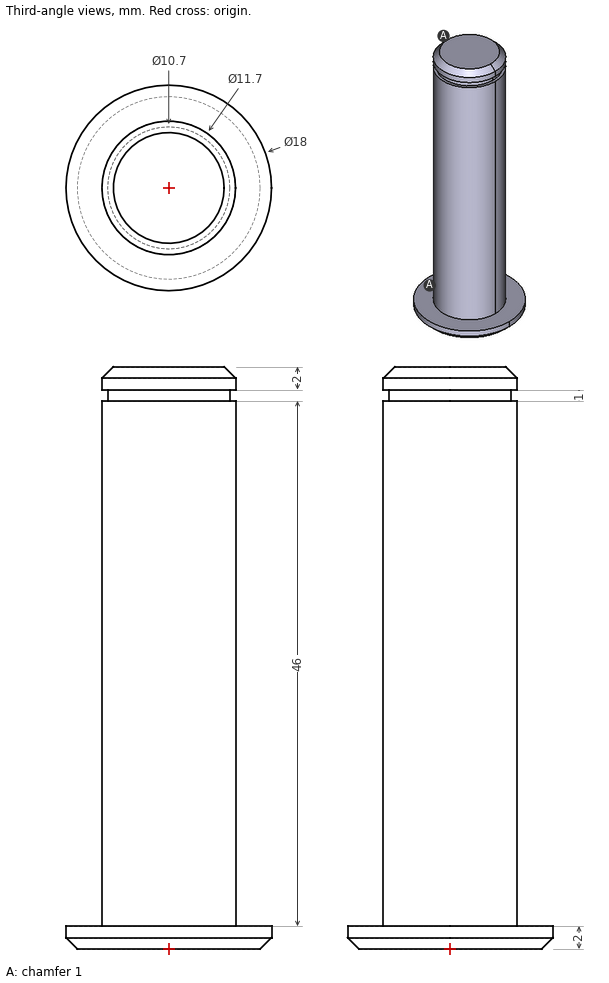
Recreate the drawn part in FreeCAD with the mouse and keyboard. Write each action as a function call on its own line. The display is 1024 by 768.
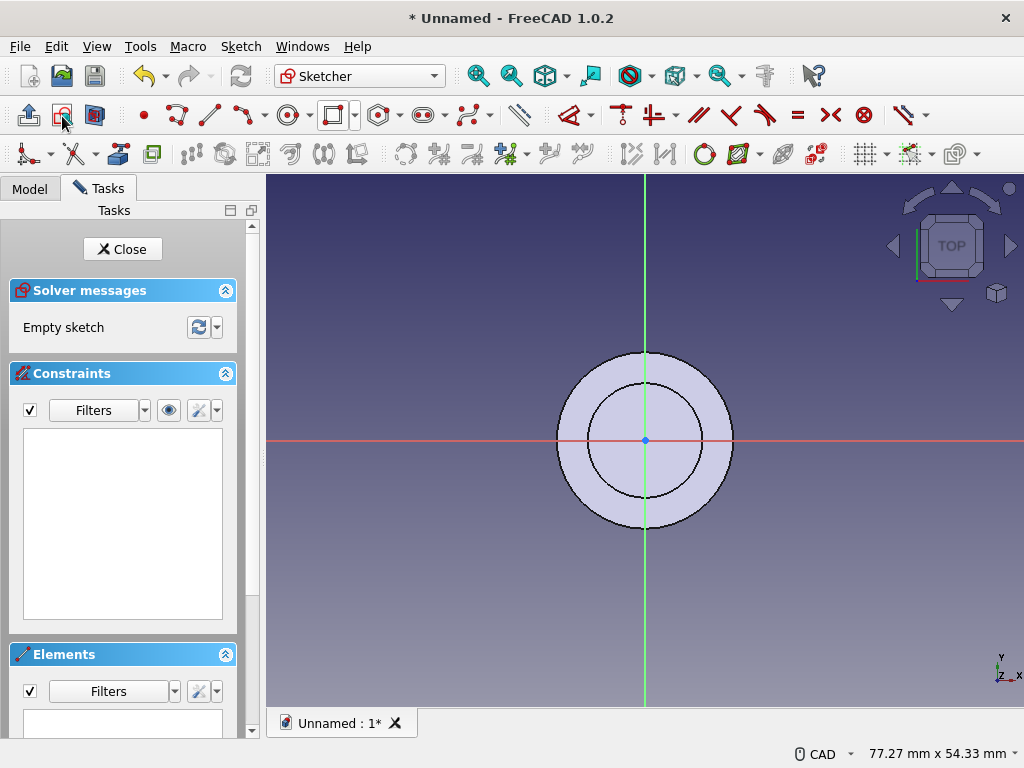
scroll(675, 440, up, 6)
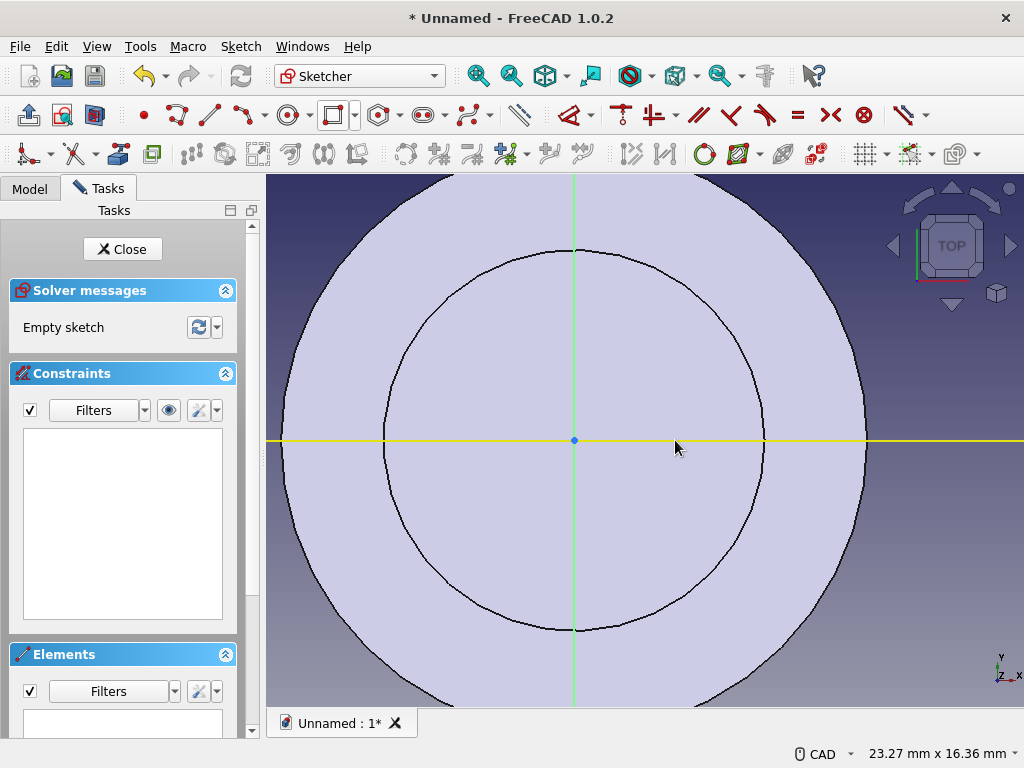
click(288, 116)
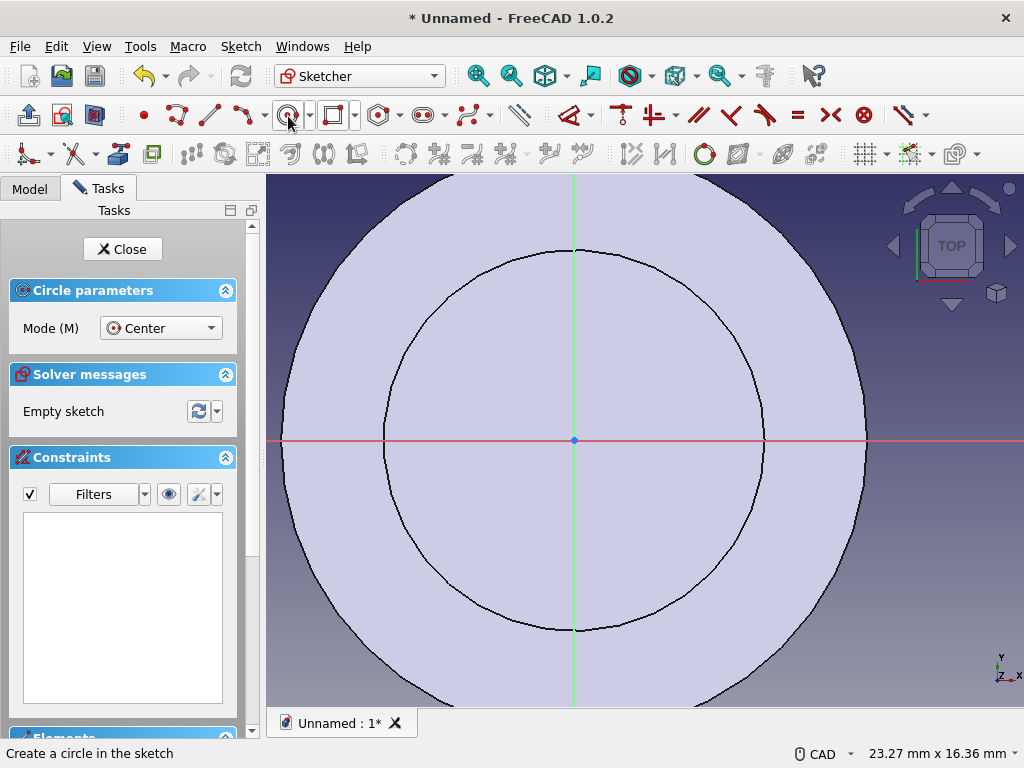
click(574, 440)
move(697, 317)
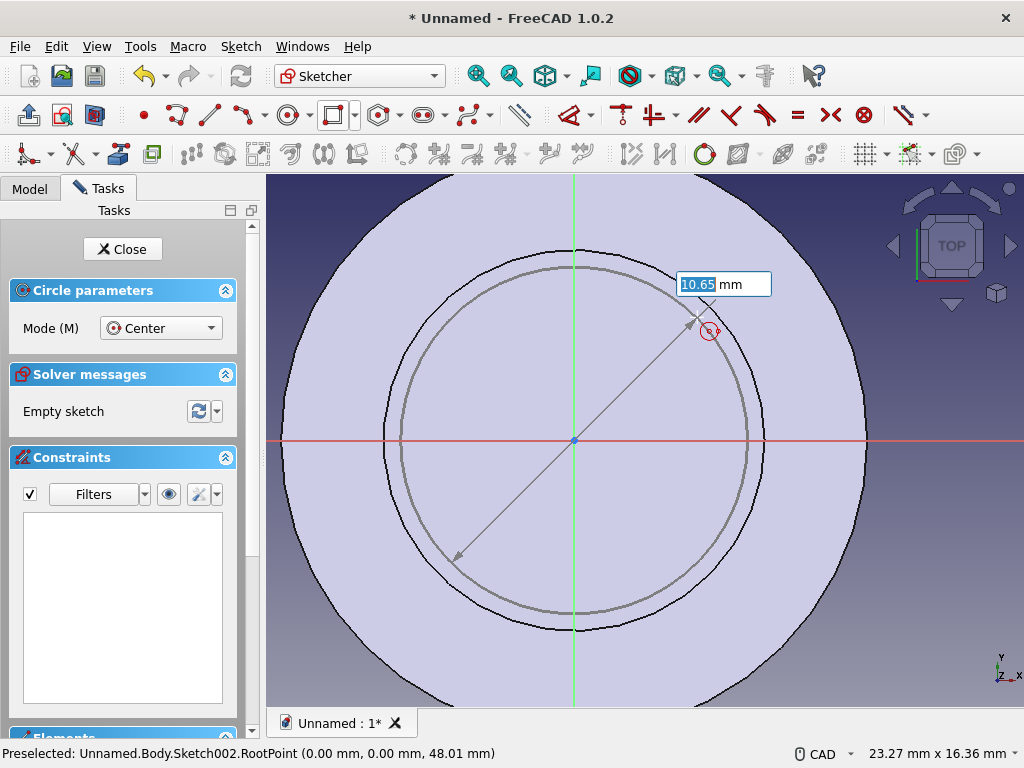
text(10.7)
key(Return)
key(Escape)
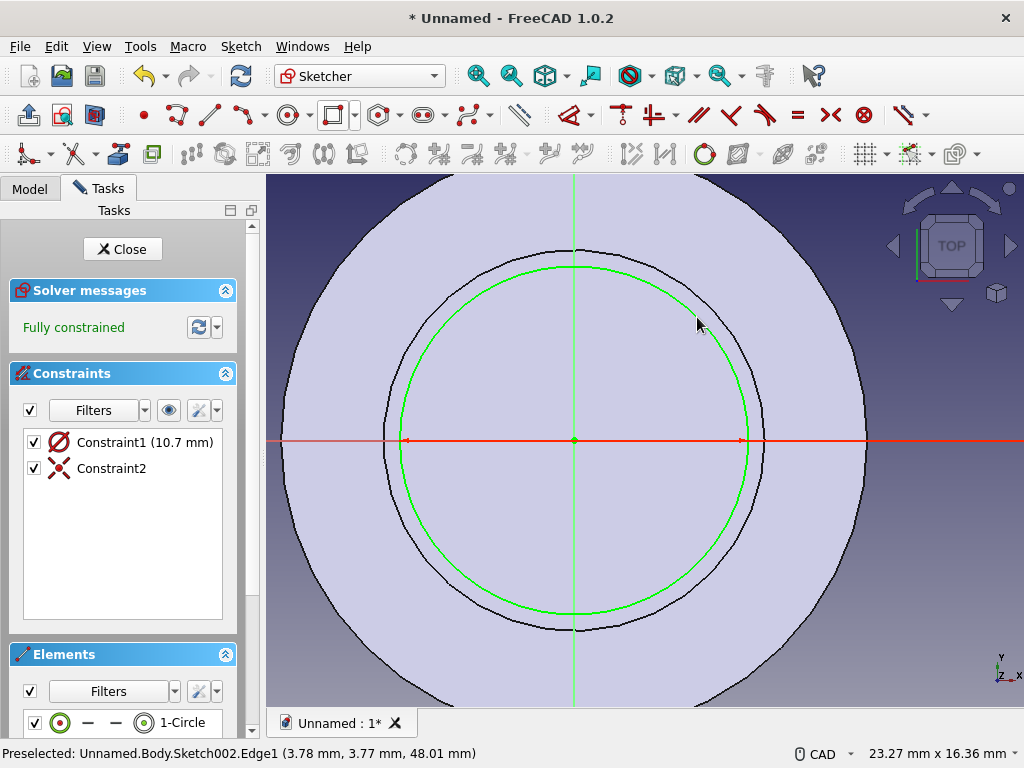
click(123, 249)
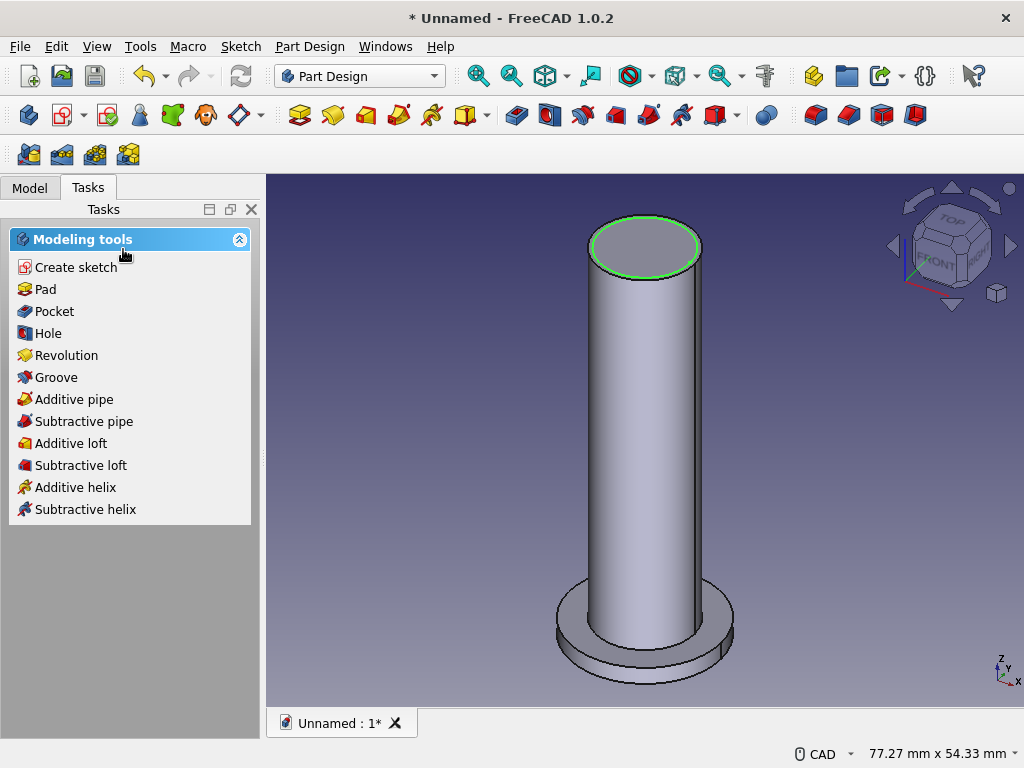
click(300, 116)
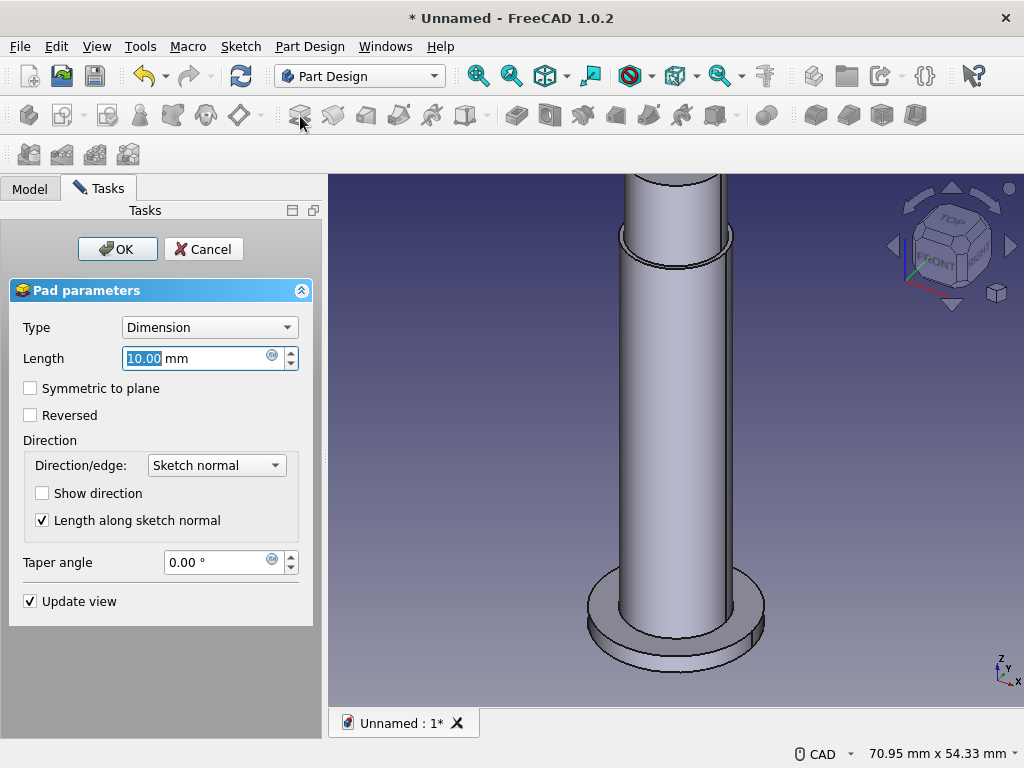
text(1)
key(Tab)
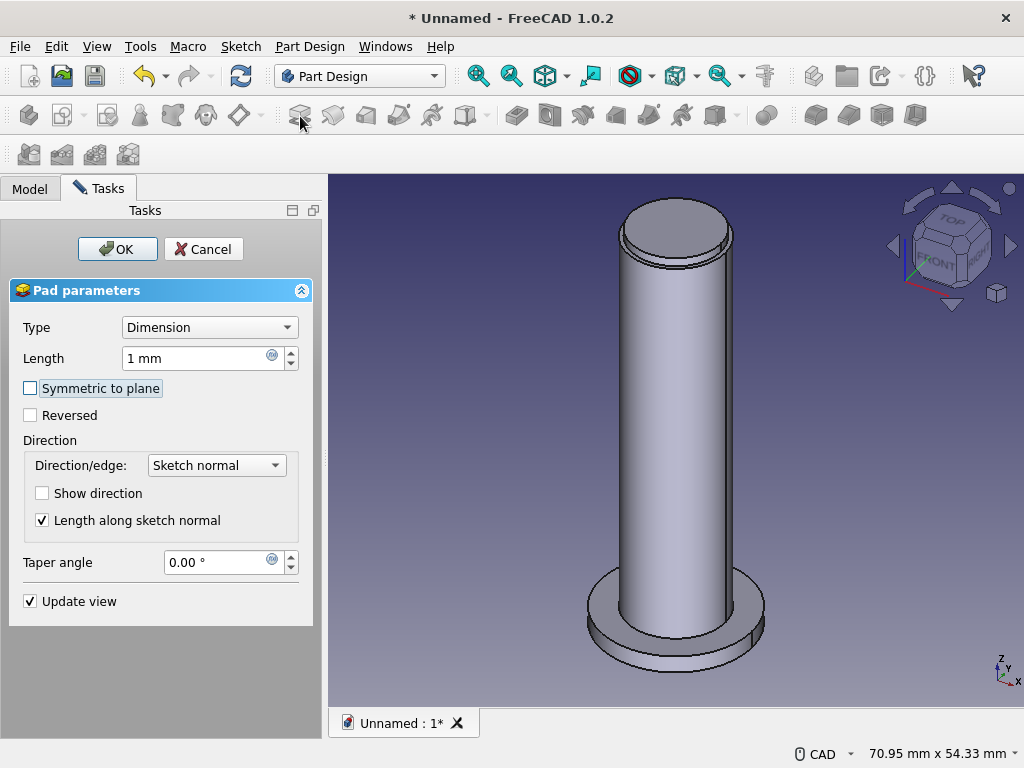
click(118, 249)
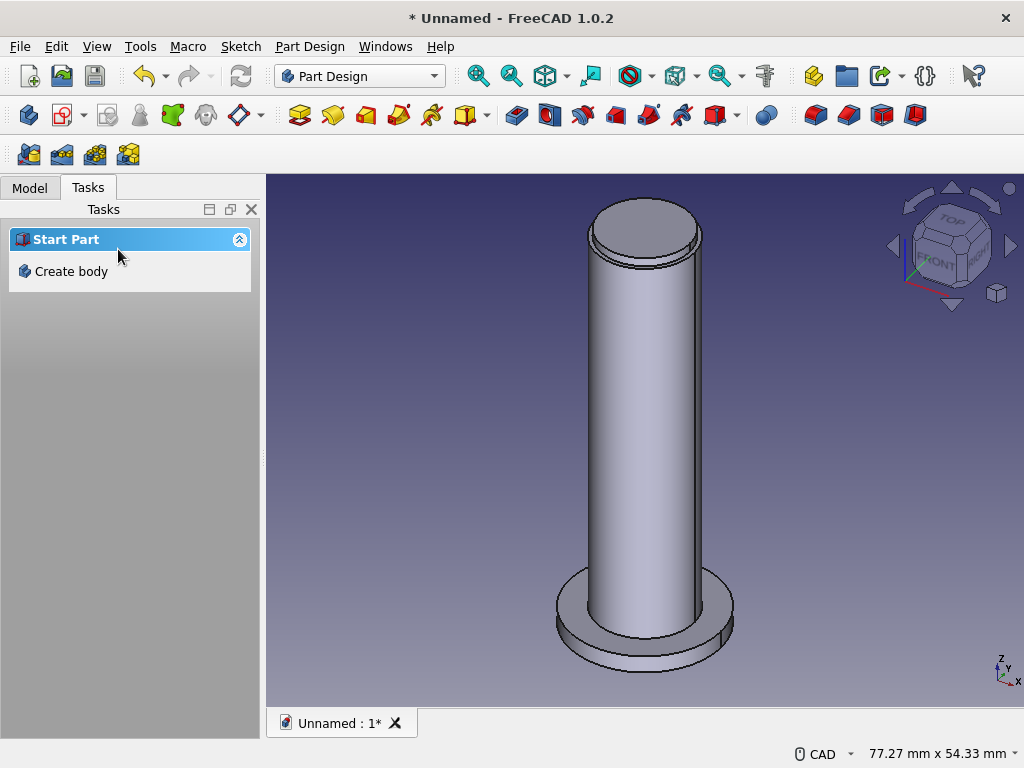
click(479, 76)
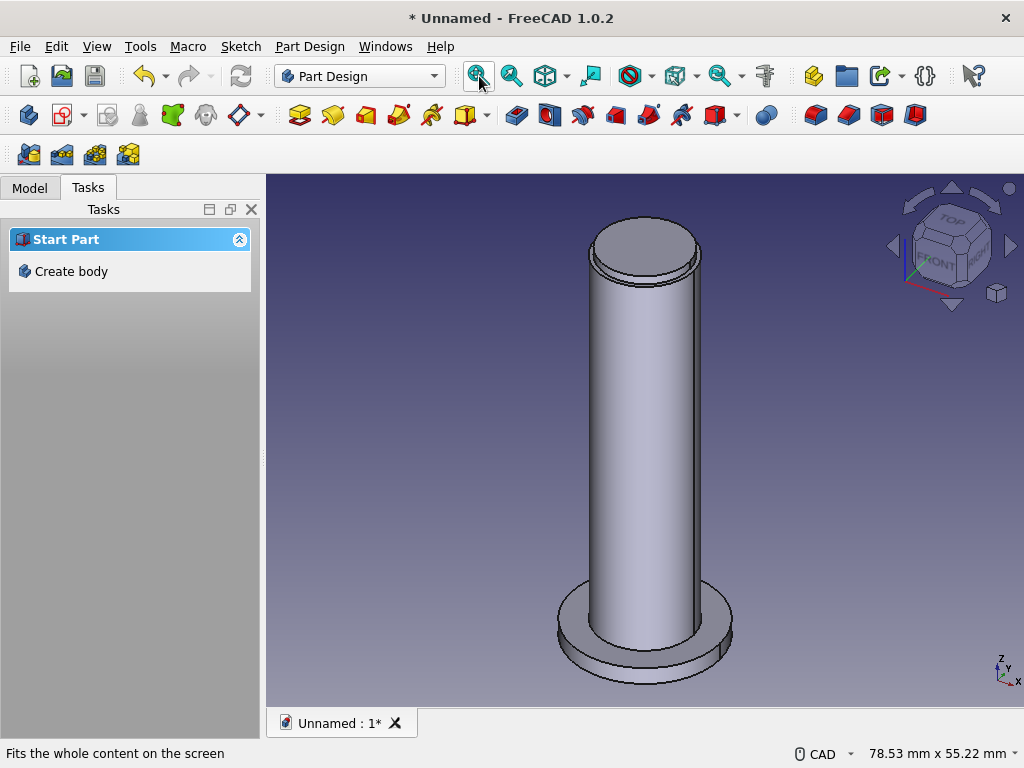
click(645, 246)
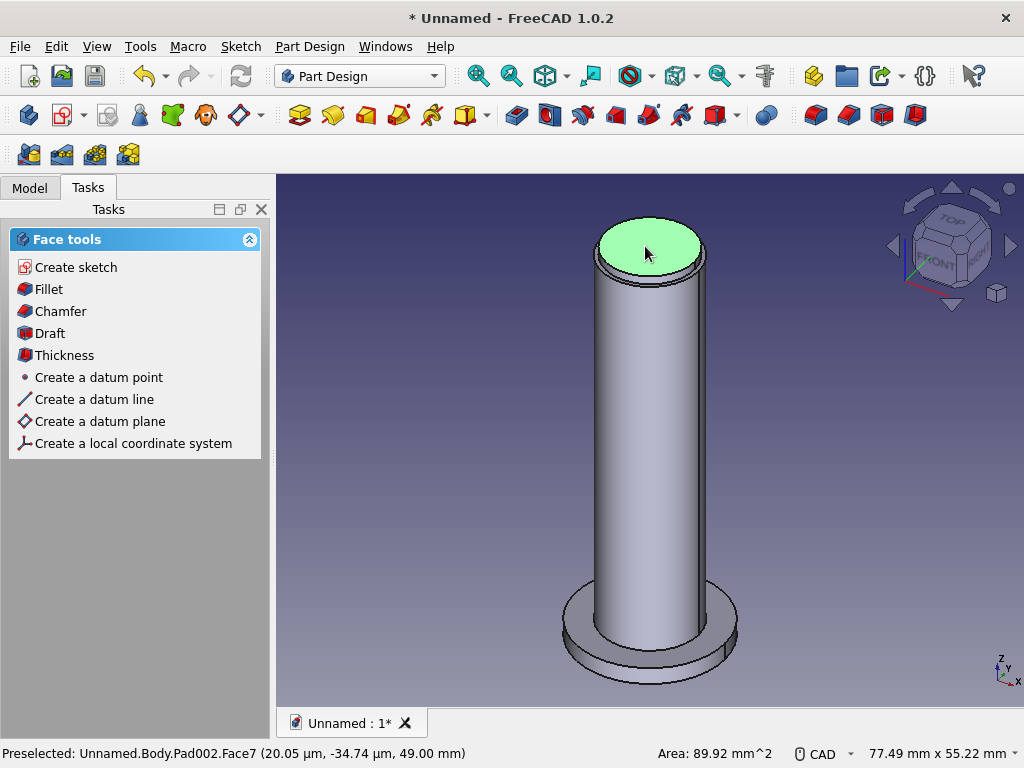
click(62, 116)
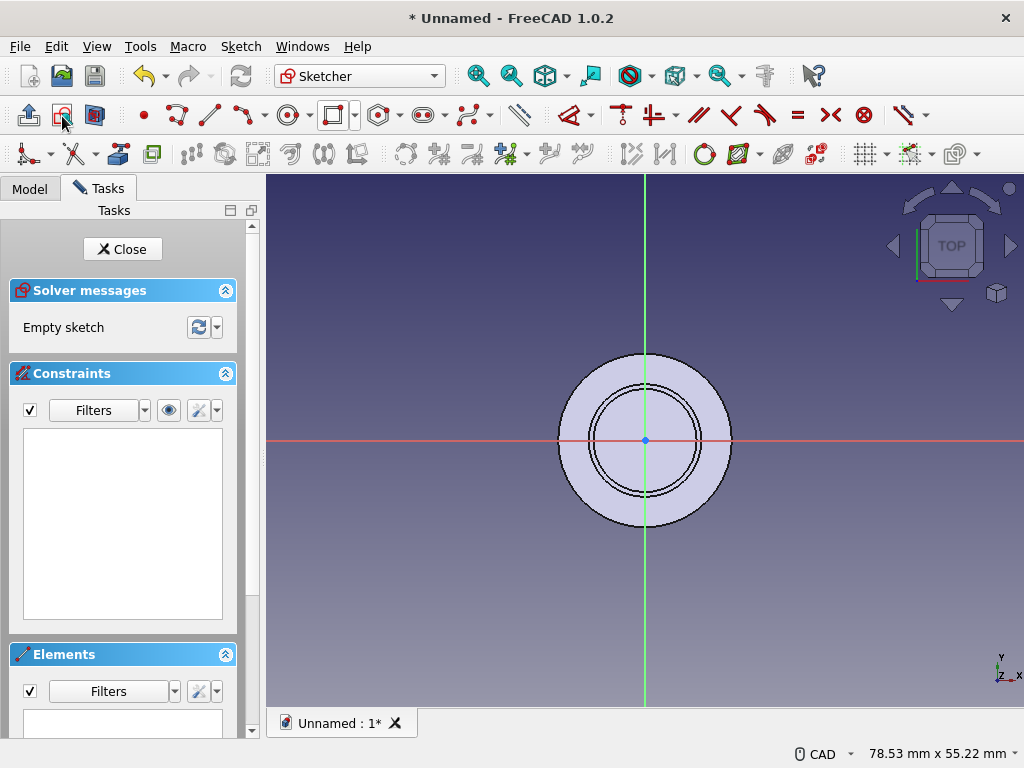
scroll(685, 440, up, 5)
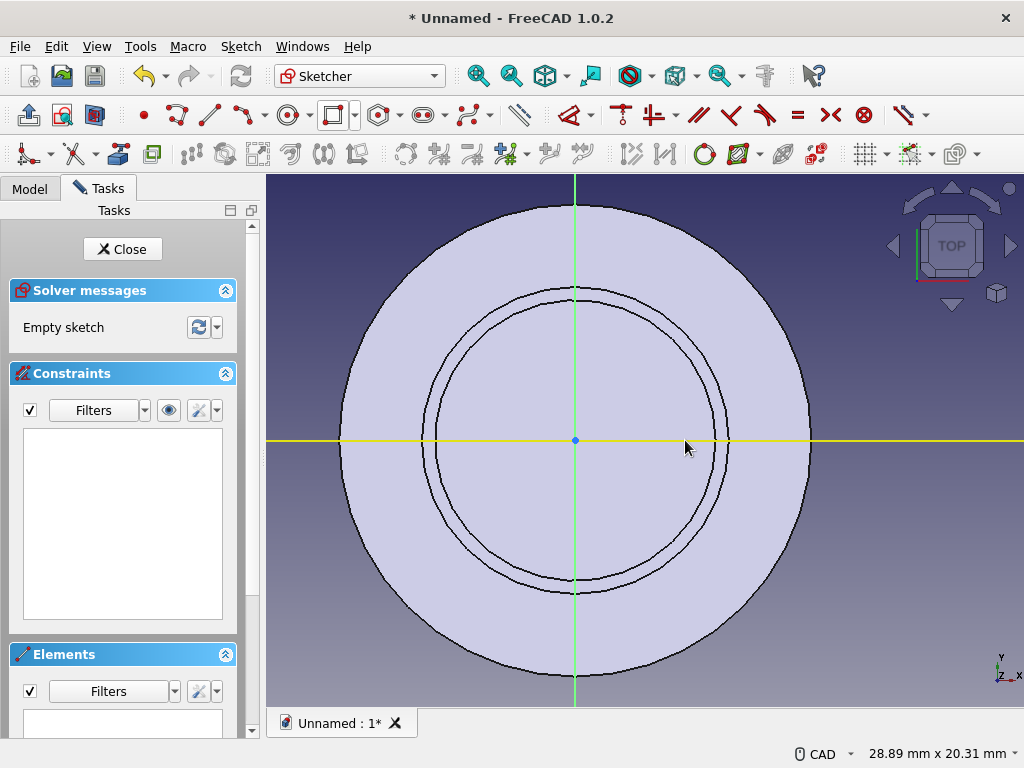
click(288, 116)